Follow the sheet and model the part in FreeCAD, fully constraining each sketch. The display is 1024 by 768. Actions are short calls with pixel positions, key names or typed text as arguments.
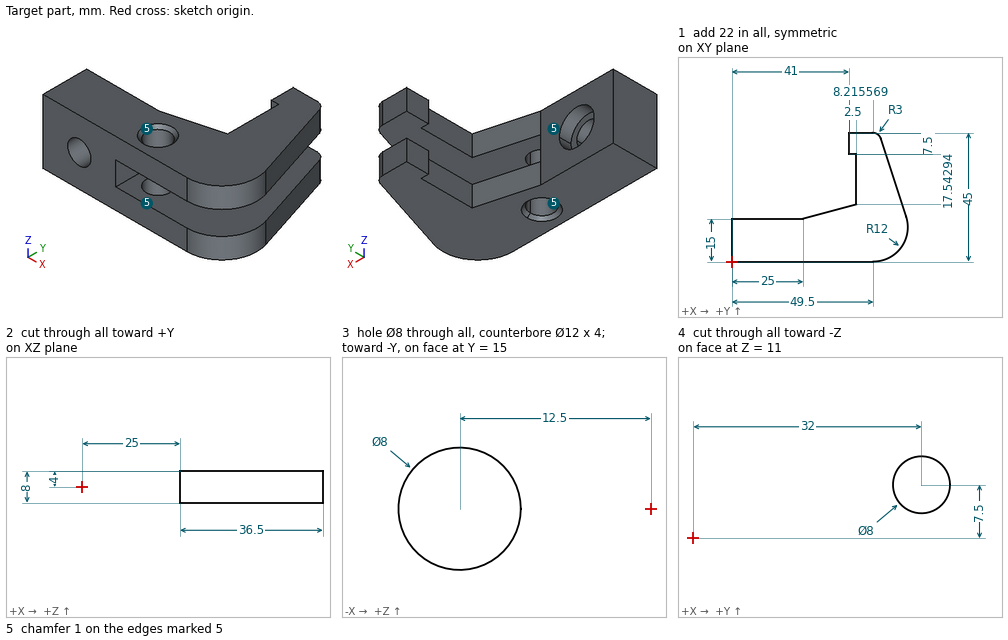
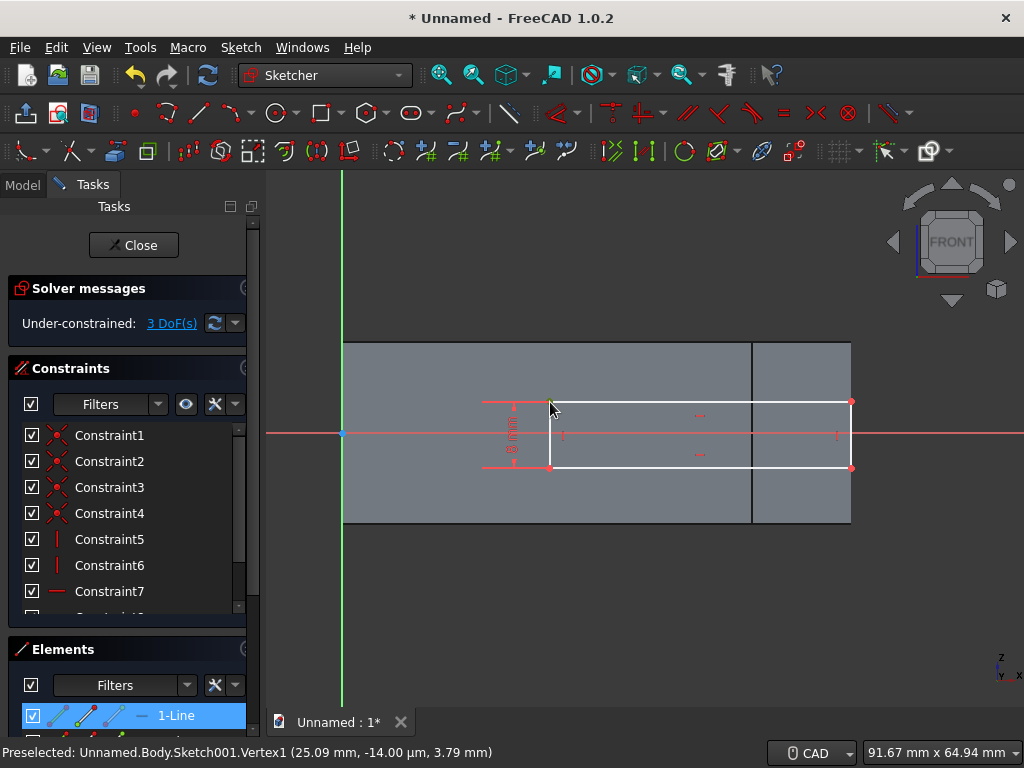
key(i)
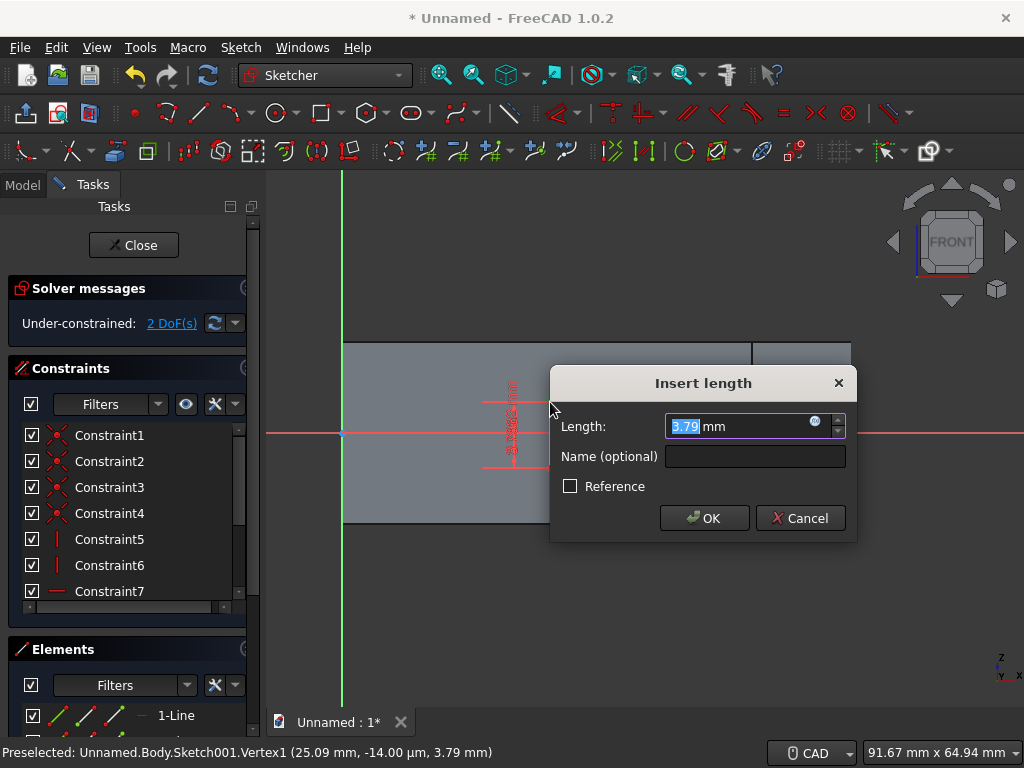
text(4)
key(Return)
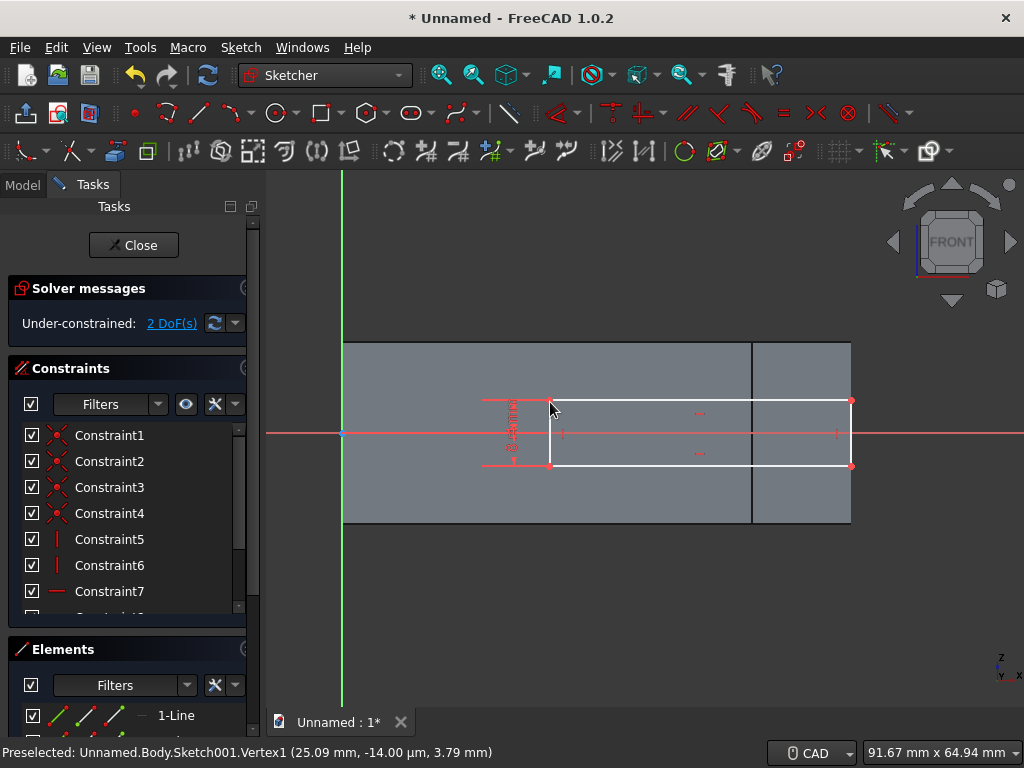
click(550, 400)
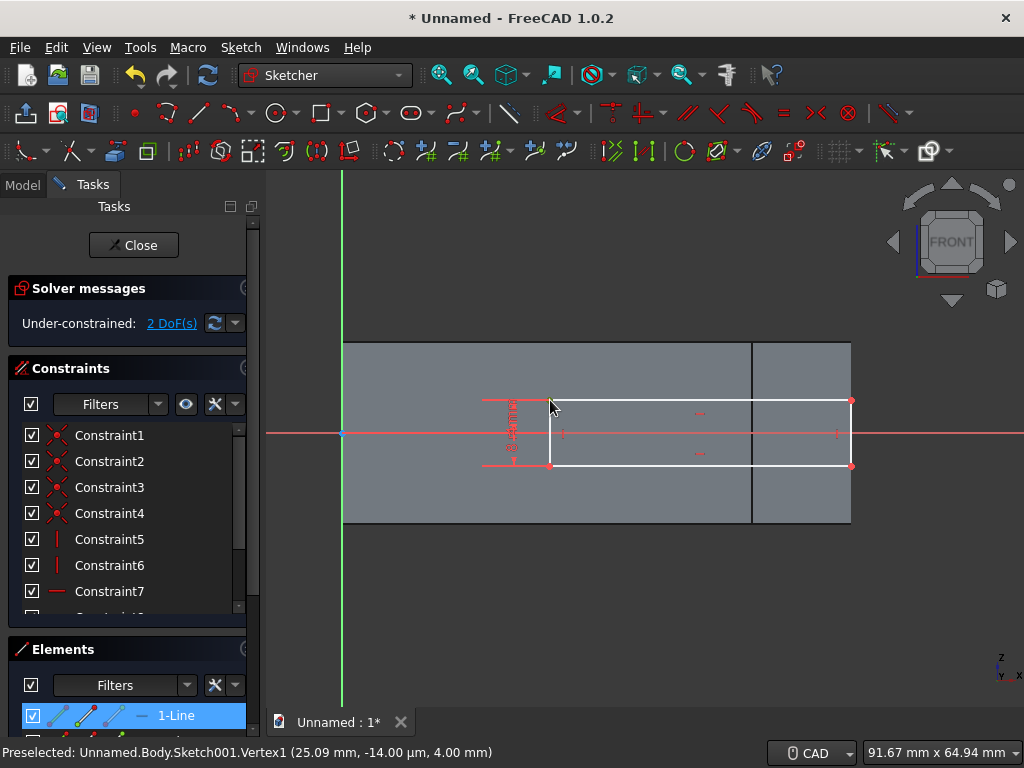
click(580, 114)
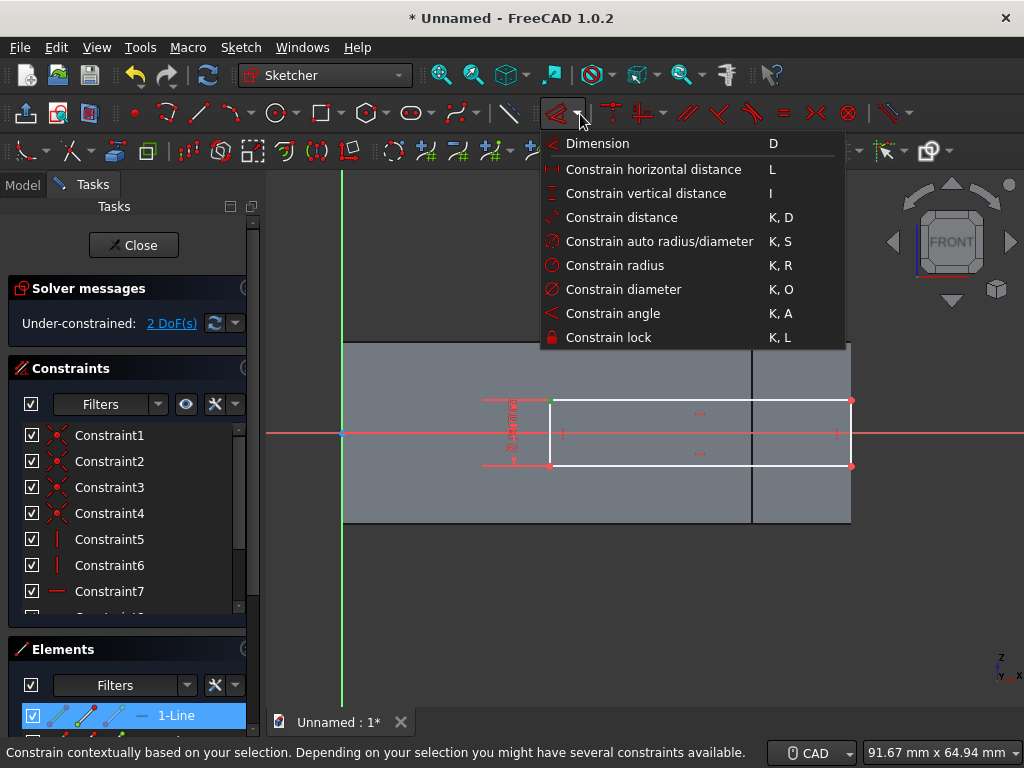
click(693, 169)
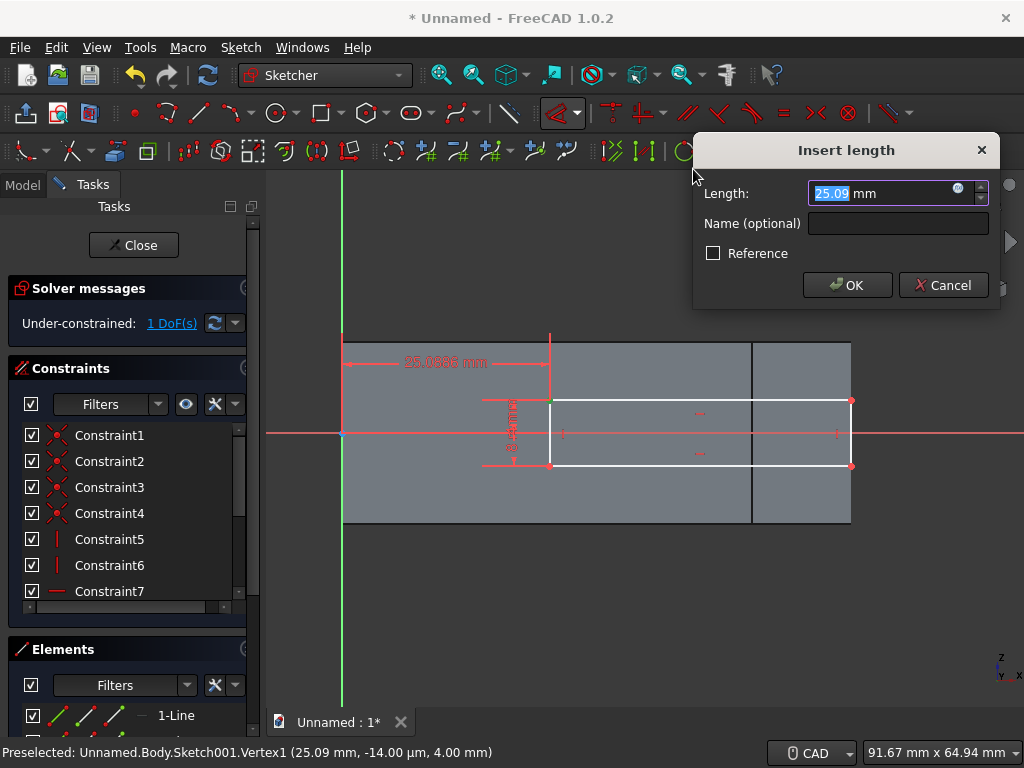
text(25)
key(Return)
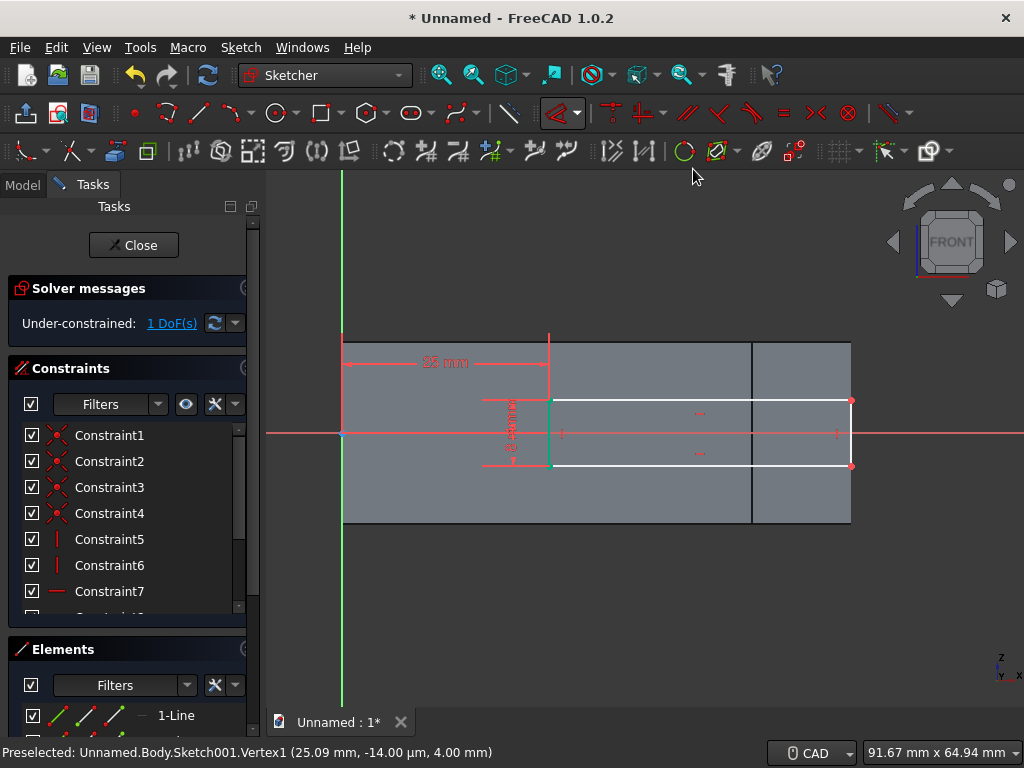
click(640, 466)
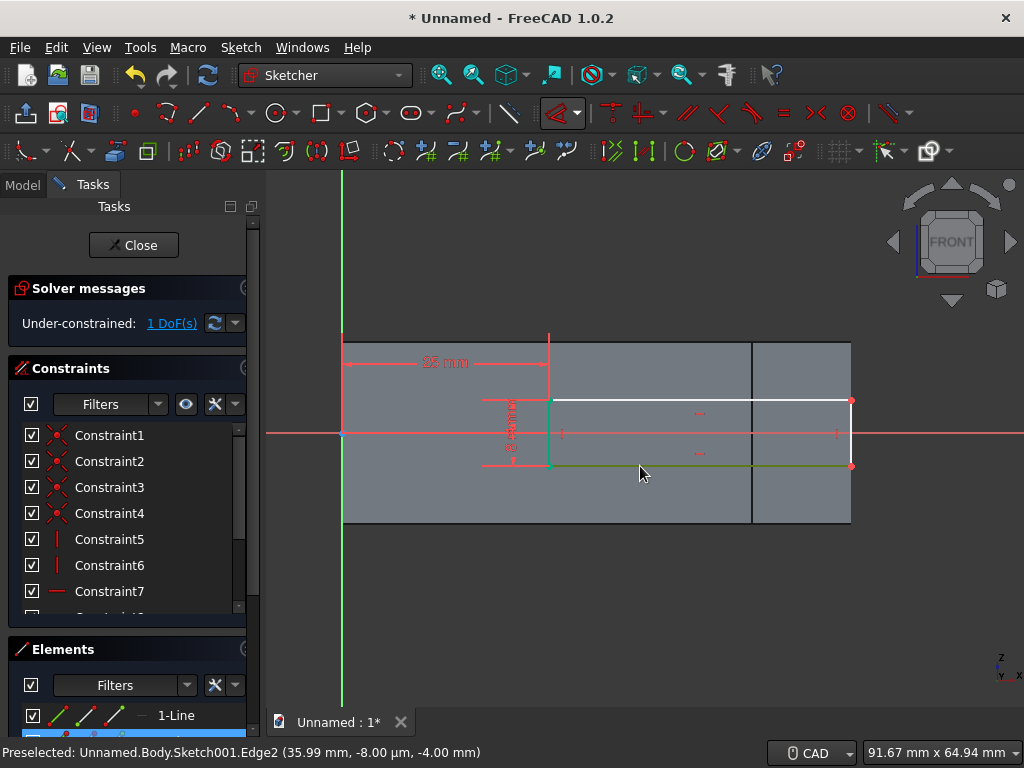
click(580, 114)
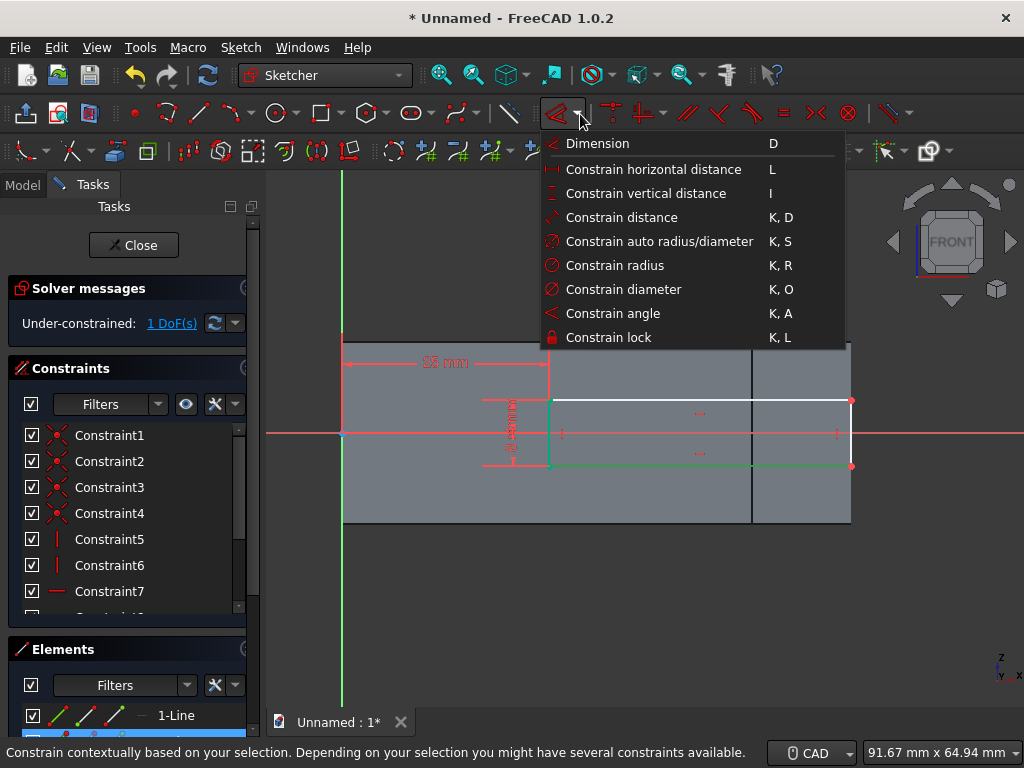
click(693, 169)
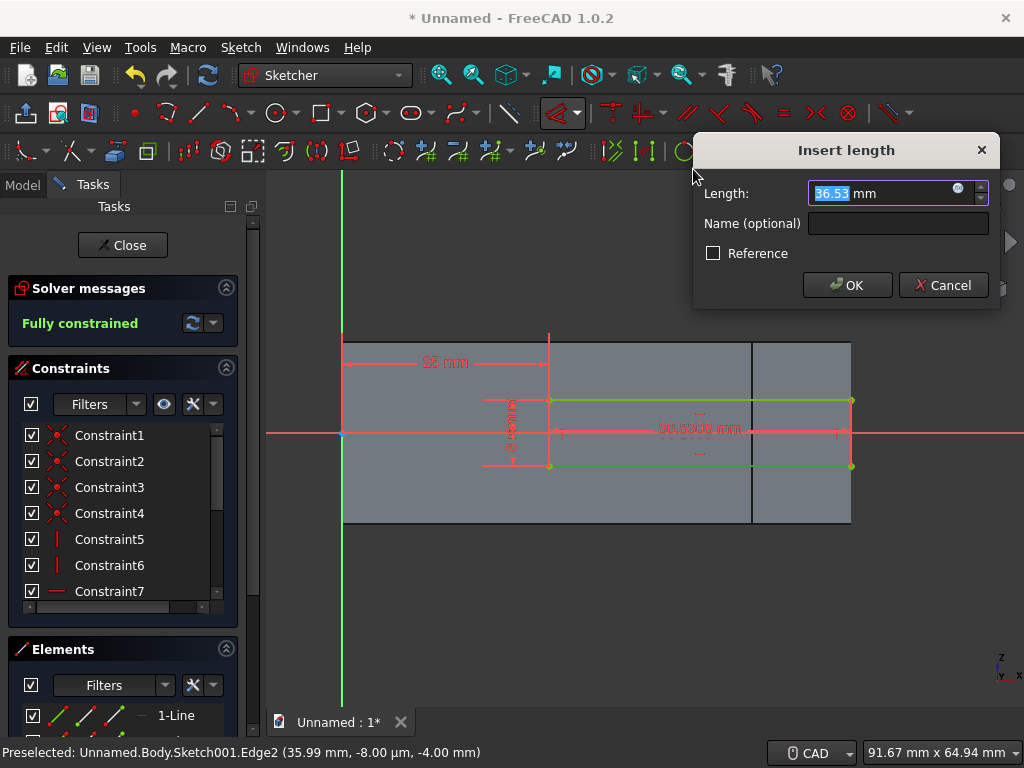
text(36.5)
key(Return)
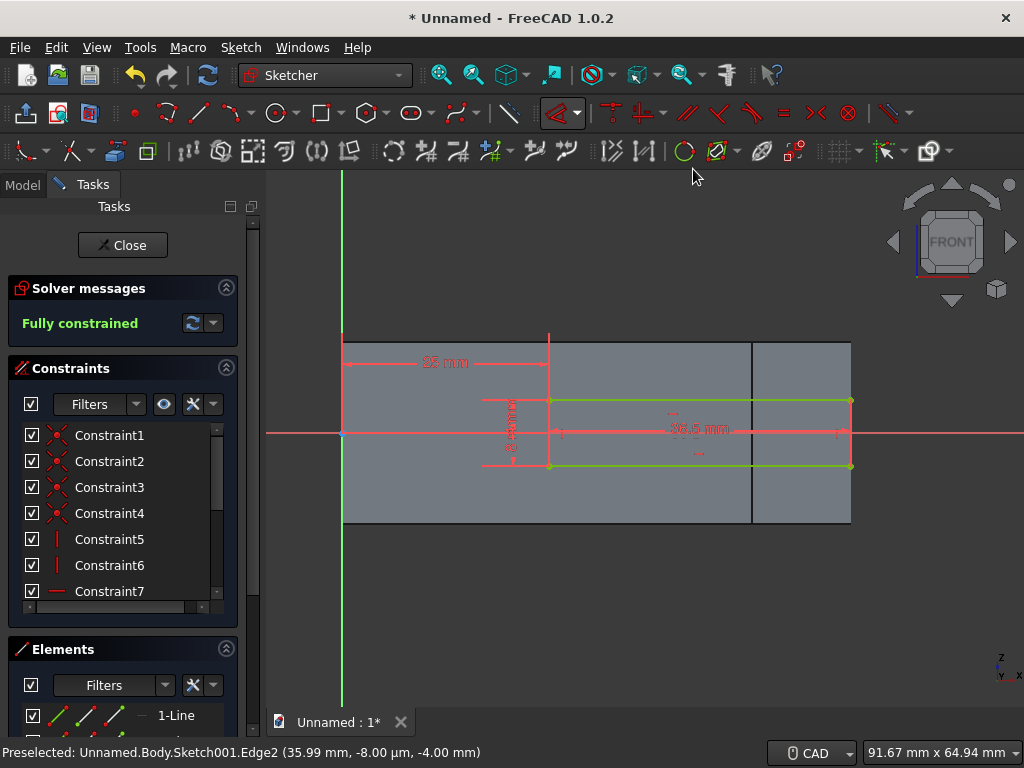
click(123, 245)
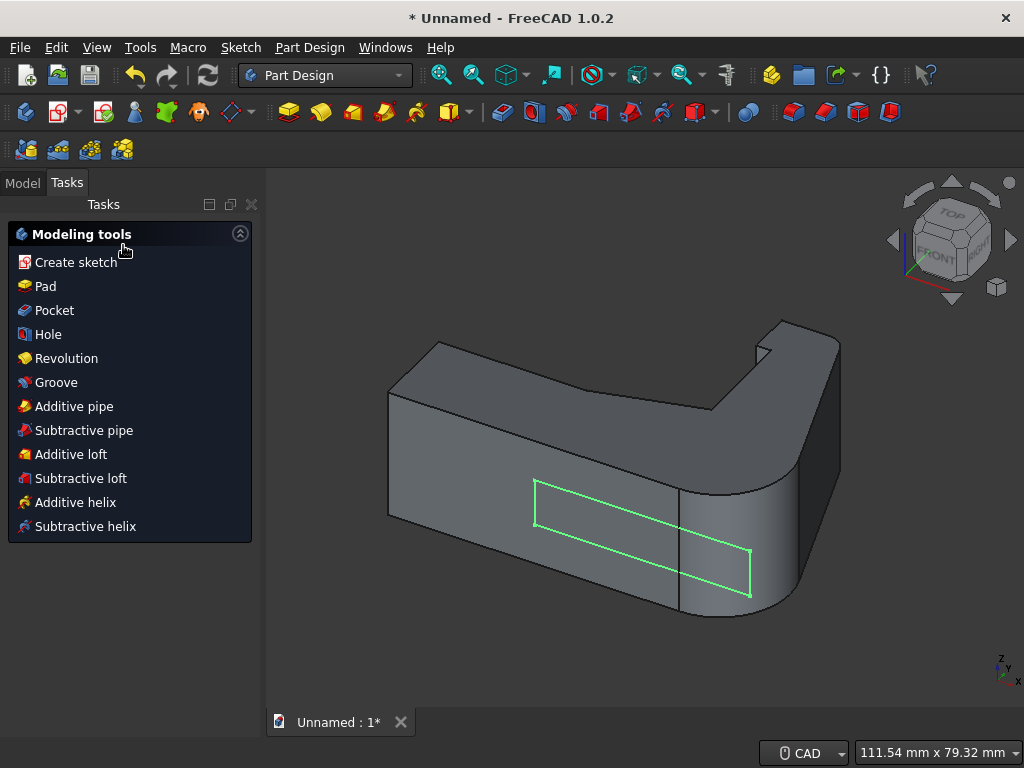
click(504, 112)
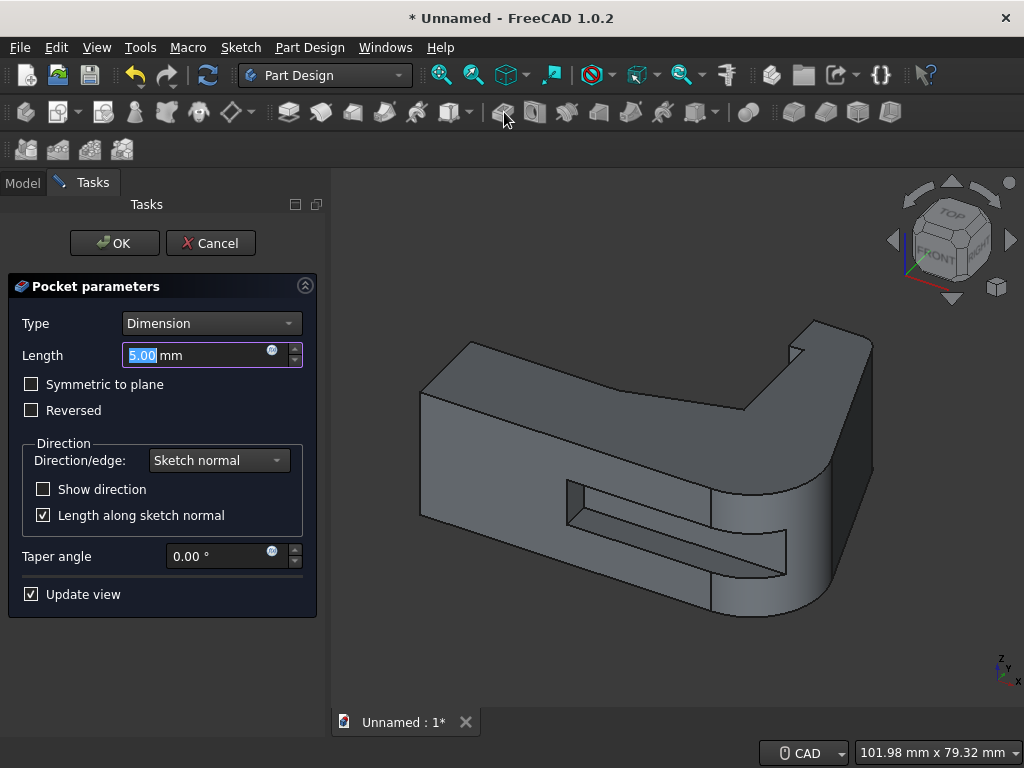
click(212, 324)